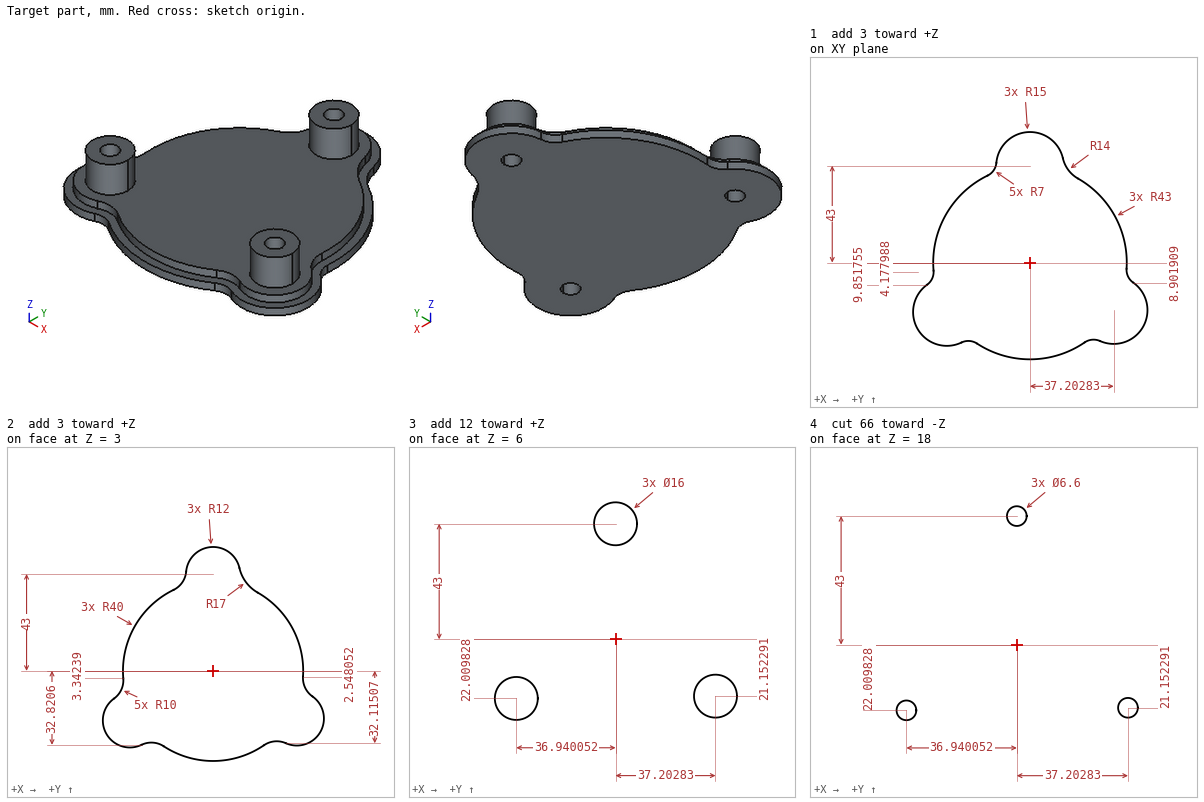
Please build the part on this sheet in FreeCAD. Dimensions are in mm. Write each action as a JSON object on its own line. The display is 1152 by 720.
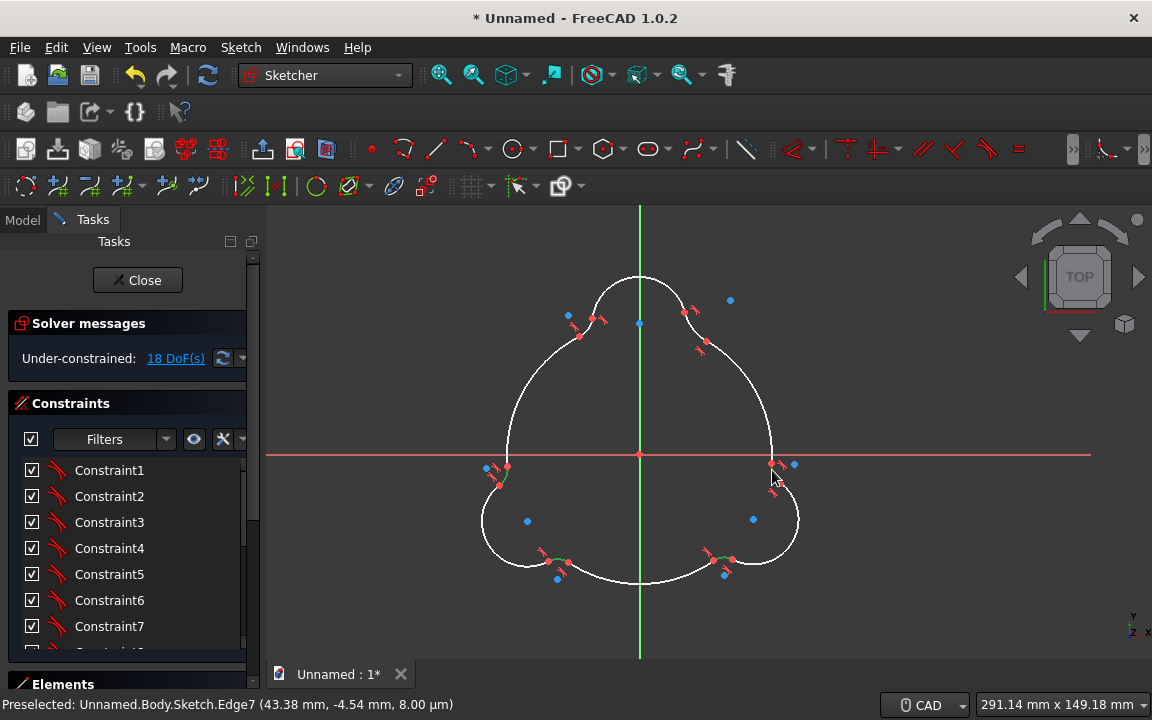
{"action": "scroll", "coordinate": [585, 333], "scroll_direction": "up", "scroll_amount": 4}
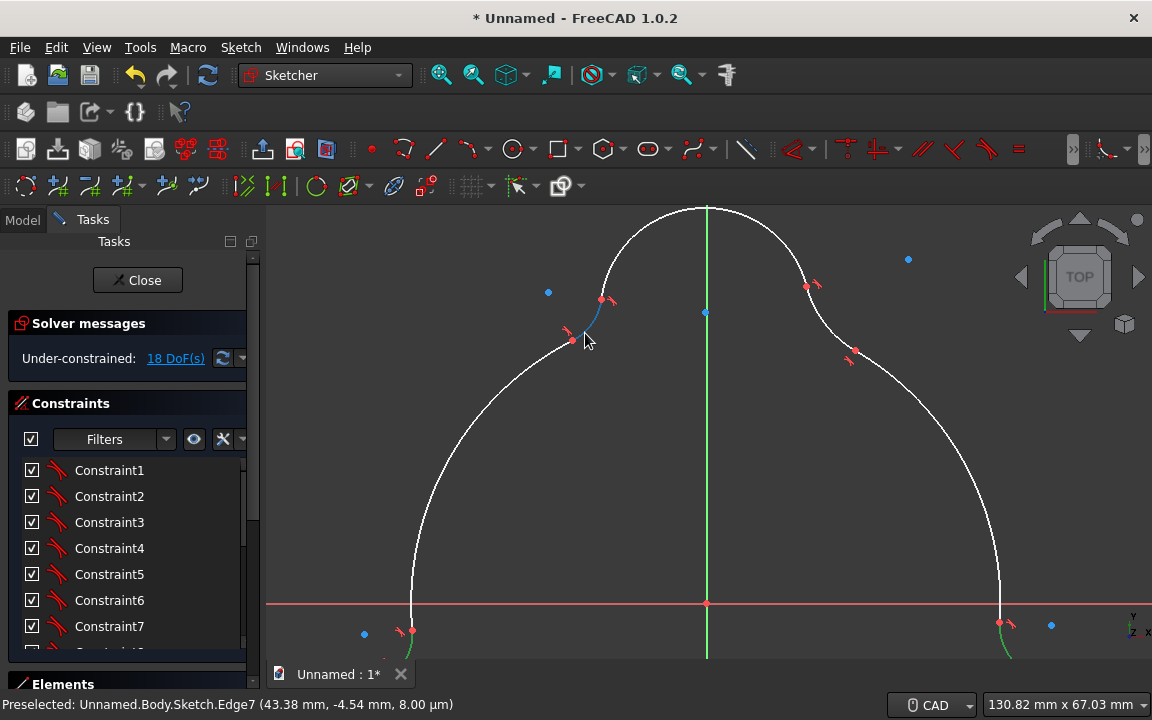
{"action": "left_click", "coordinate": [585, 332]}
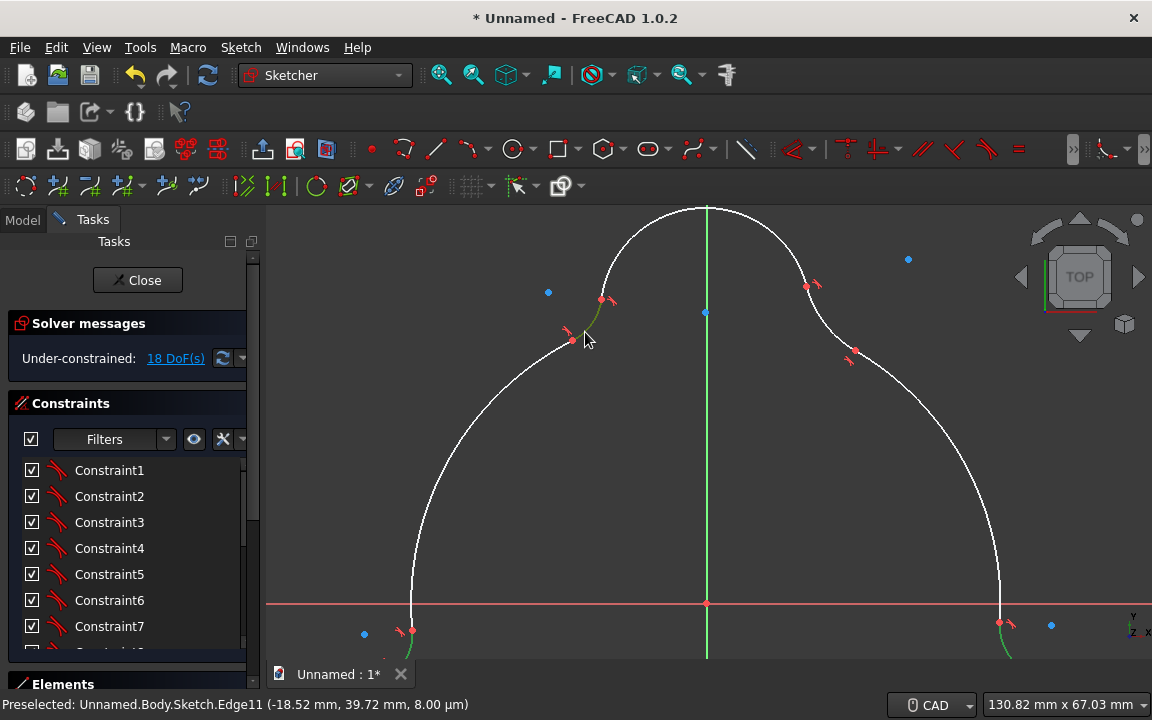
{"action": "left_click", "coordinate": [1020, 150]}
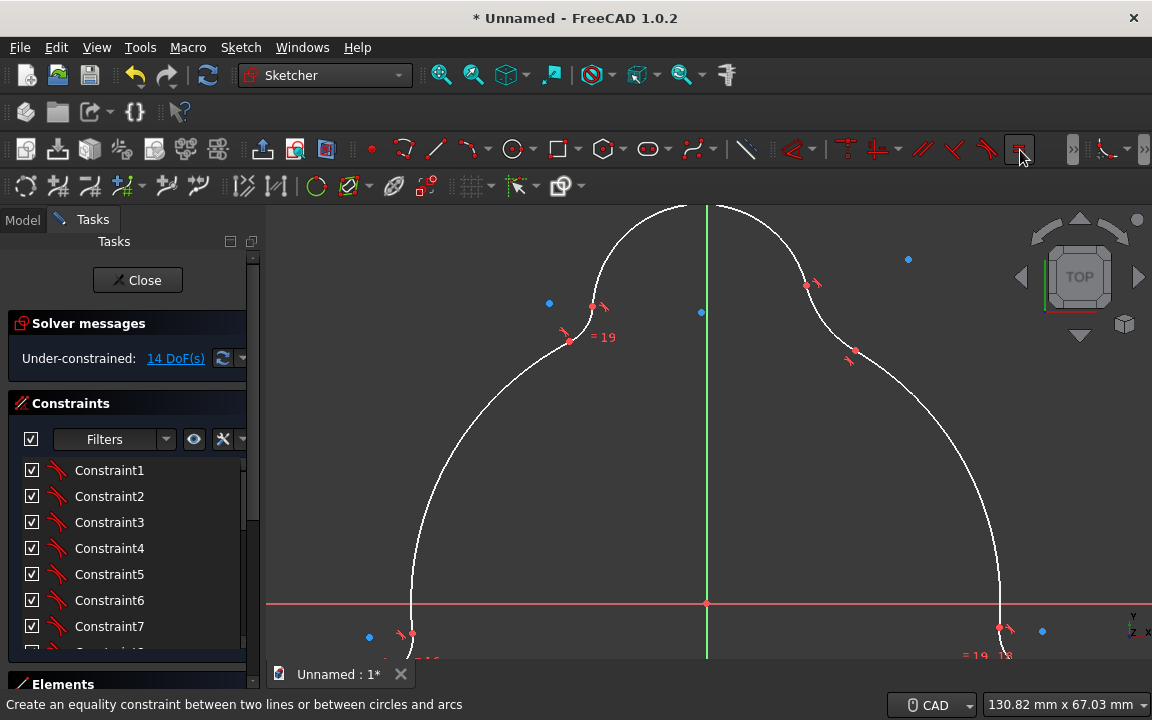
{"action": "scroll", "coordinate": [585, 333], "scroll_direction": "down", "scroll_amount": 4}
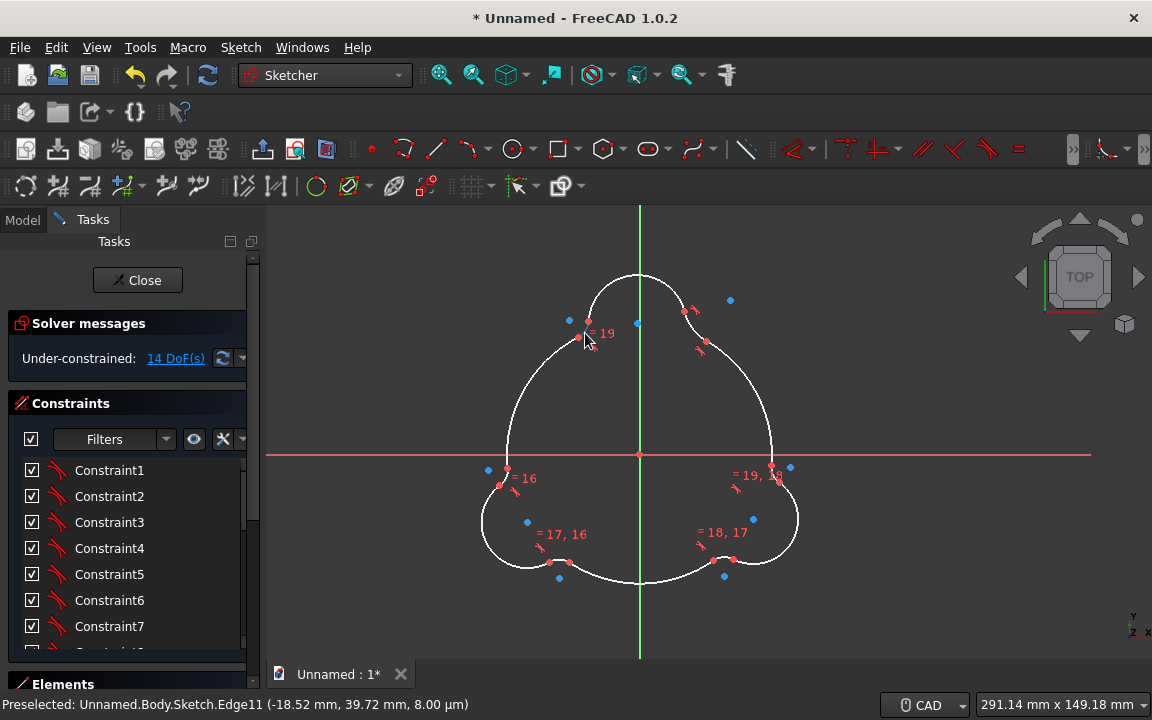
{"action": "left_click", "coordinate": [482, 521]}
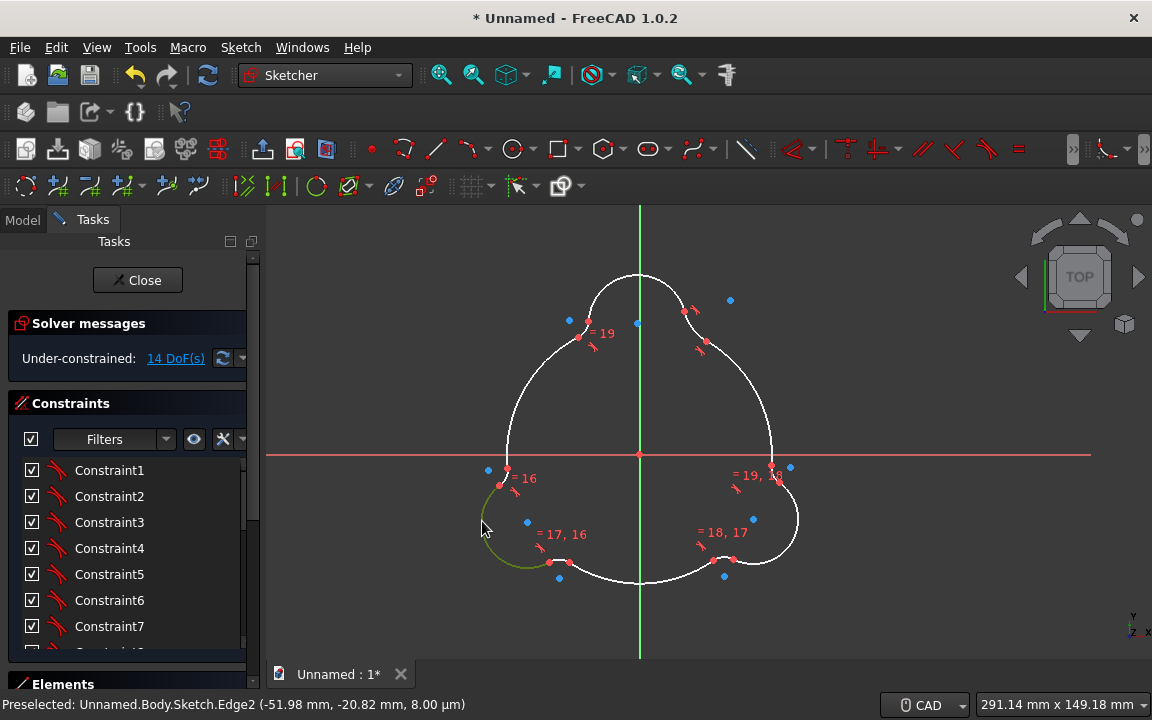
{"action": "left_click", "coordinate": [772, 560]}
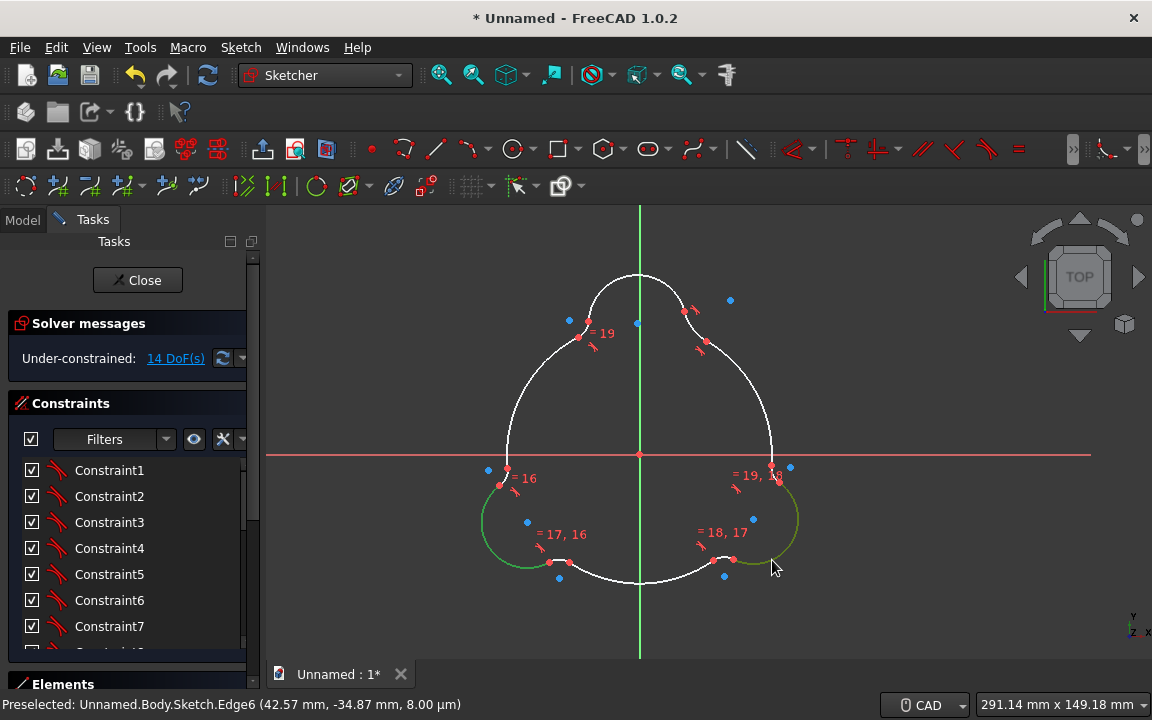
{"action": "left_click", "coordinate": [660, 281]}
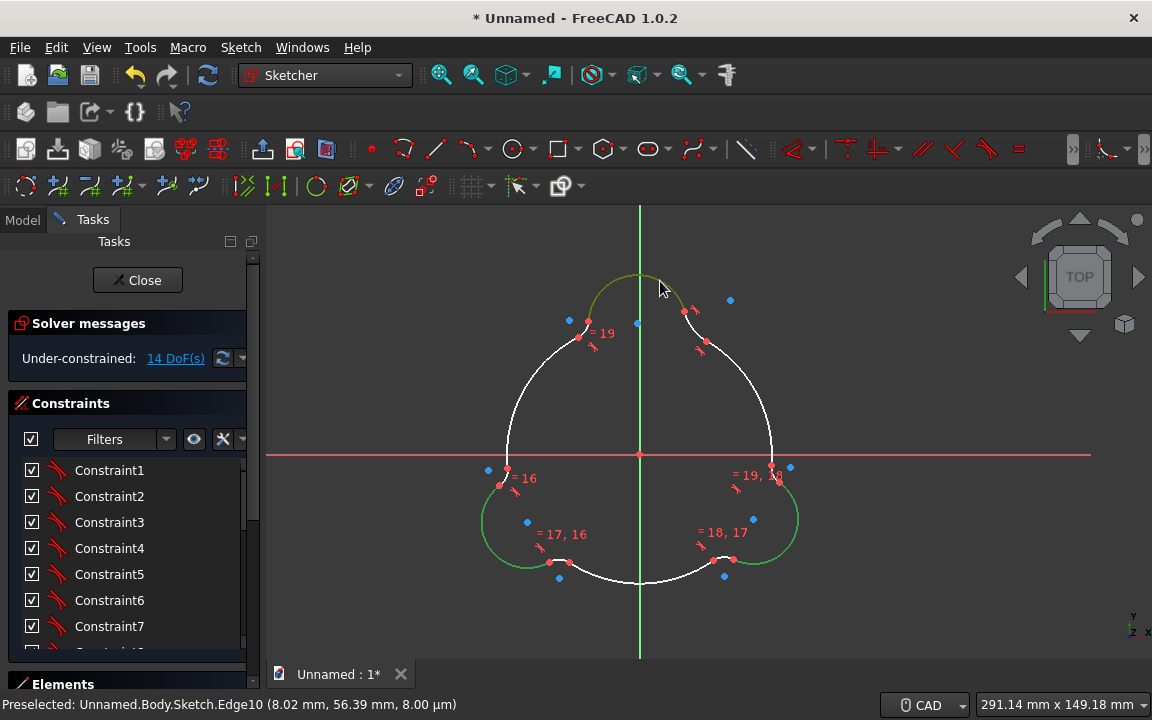
{"action": "left_click", "coordinate": [1020, 150]}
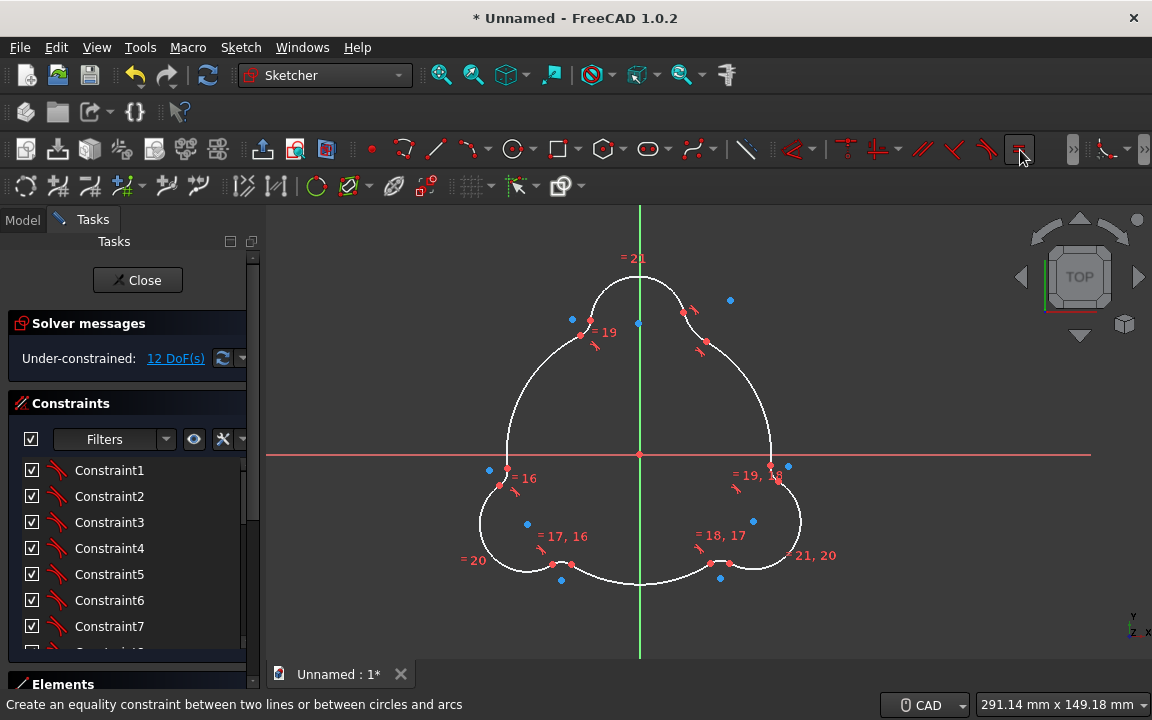
{"action": "left_click", "coordinate": [612, 582]}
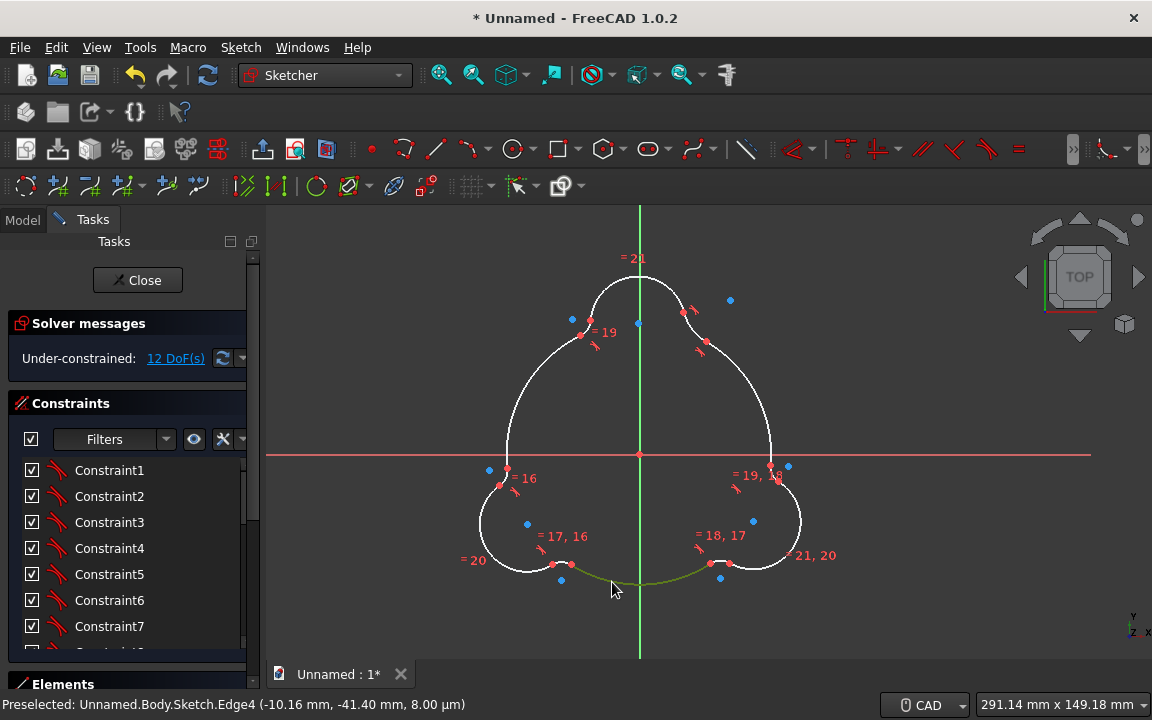
{"action": "left_click", "coordinate": [767, 422]}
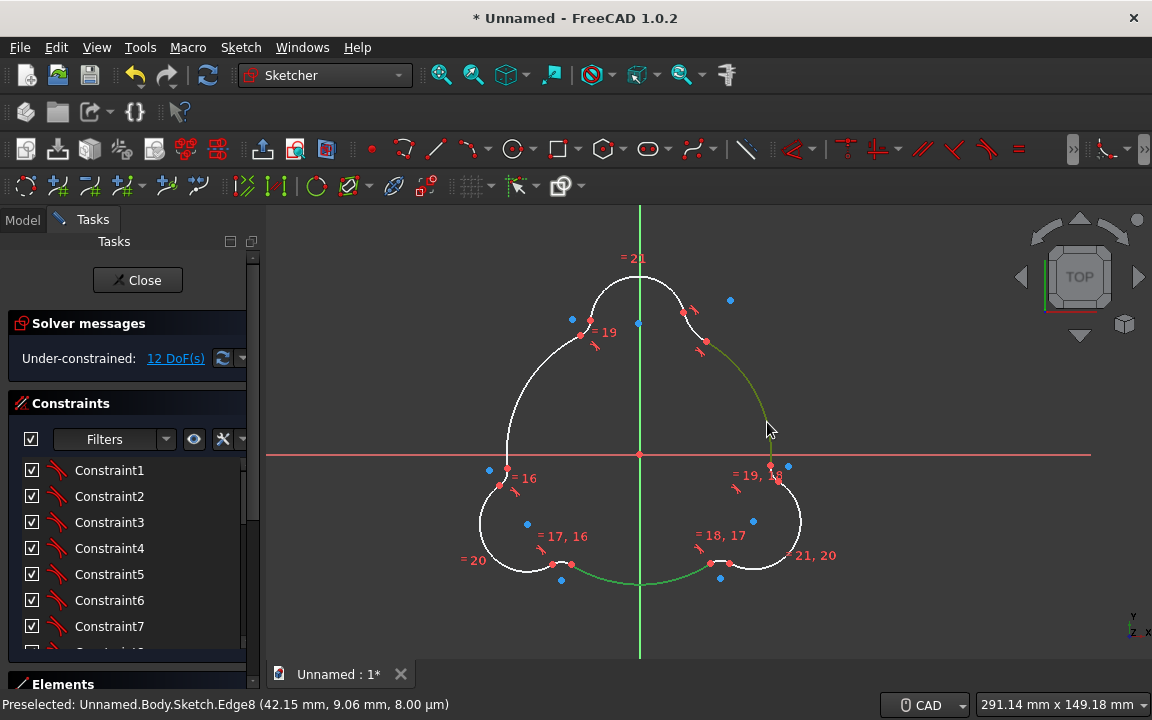
{"action": "left_click", "coordinate": [542, 364]}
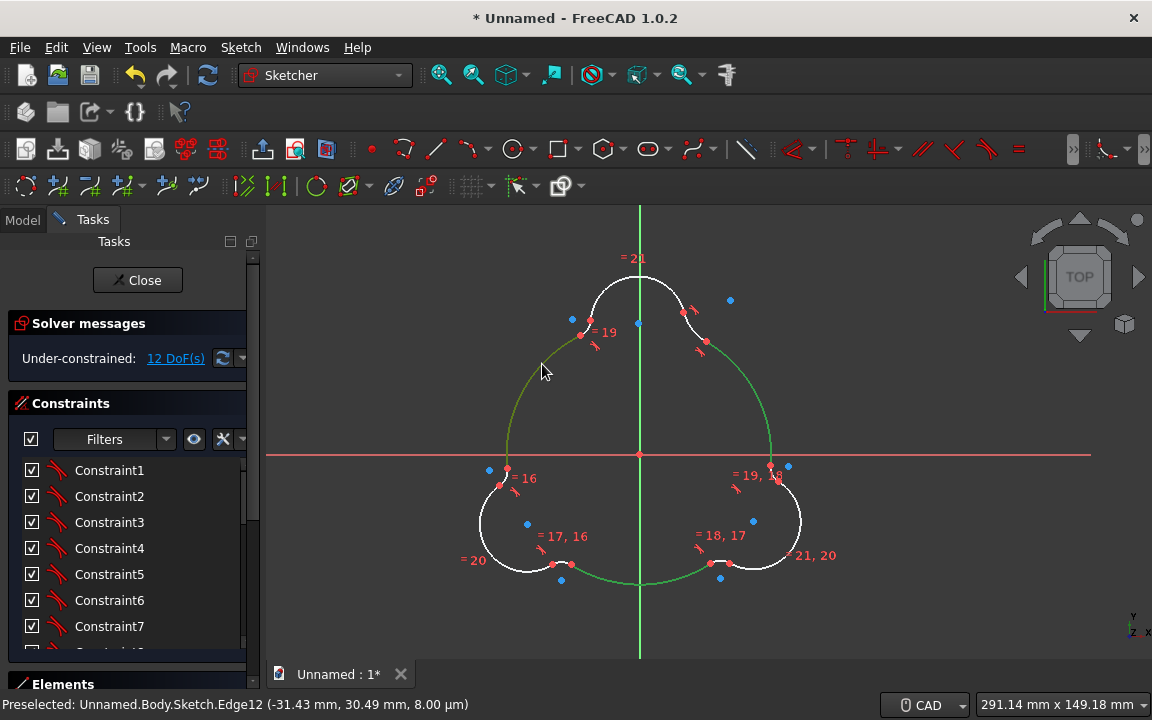
{"action": "left_click", "coordinate": [1020, 150]}